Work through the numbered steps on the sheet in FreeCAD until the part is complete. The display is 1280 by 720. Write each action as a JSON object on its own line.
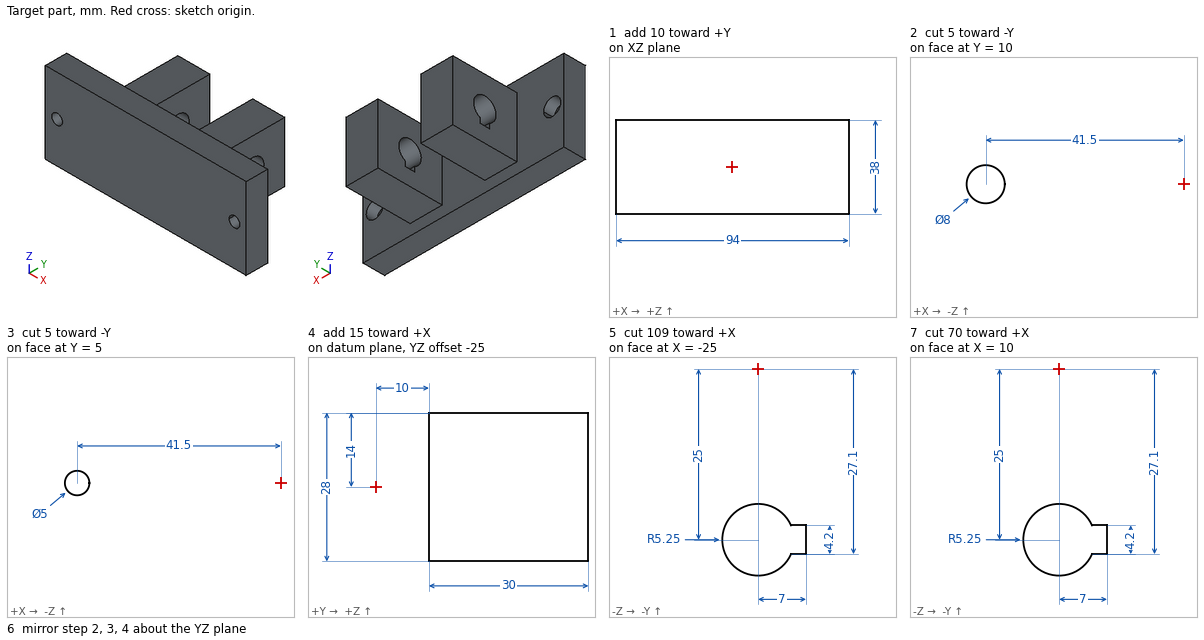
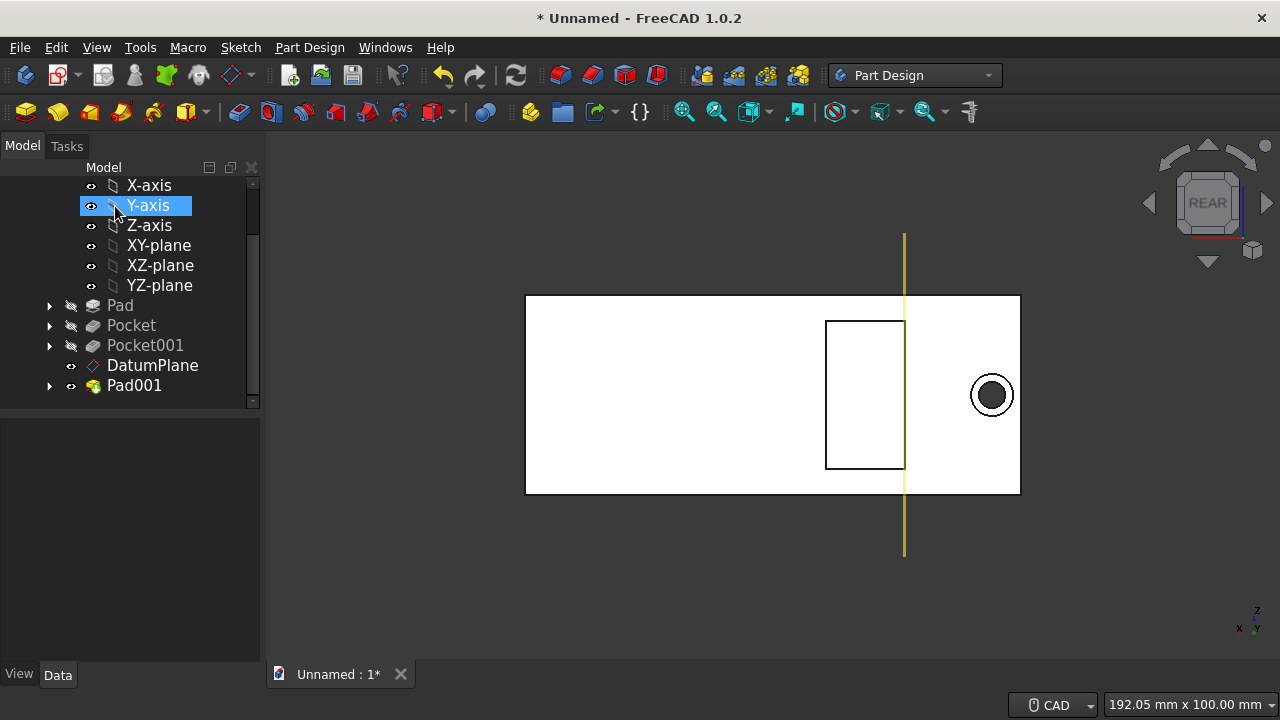
{"action": "left_click", "coordinate": [116, 366]}
{"action": "key", "text": "space"}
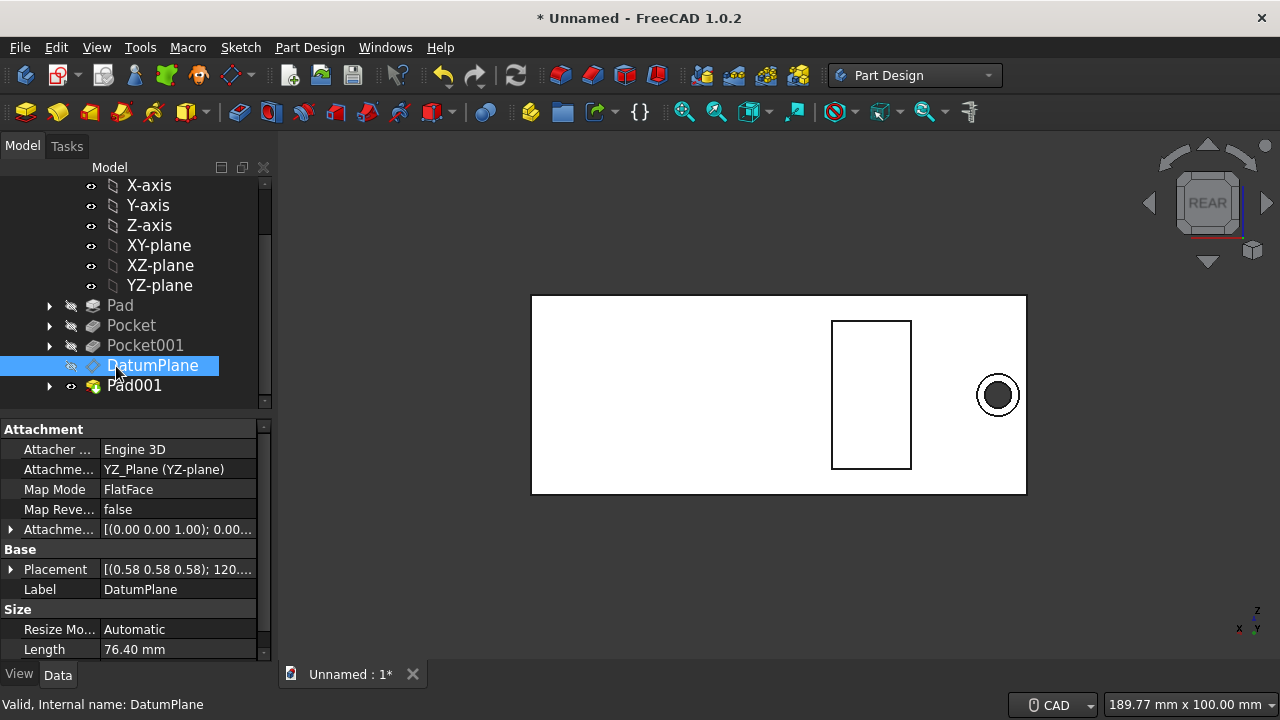
{"action": "key", "text": "6"}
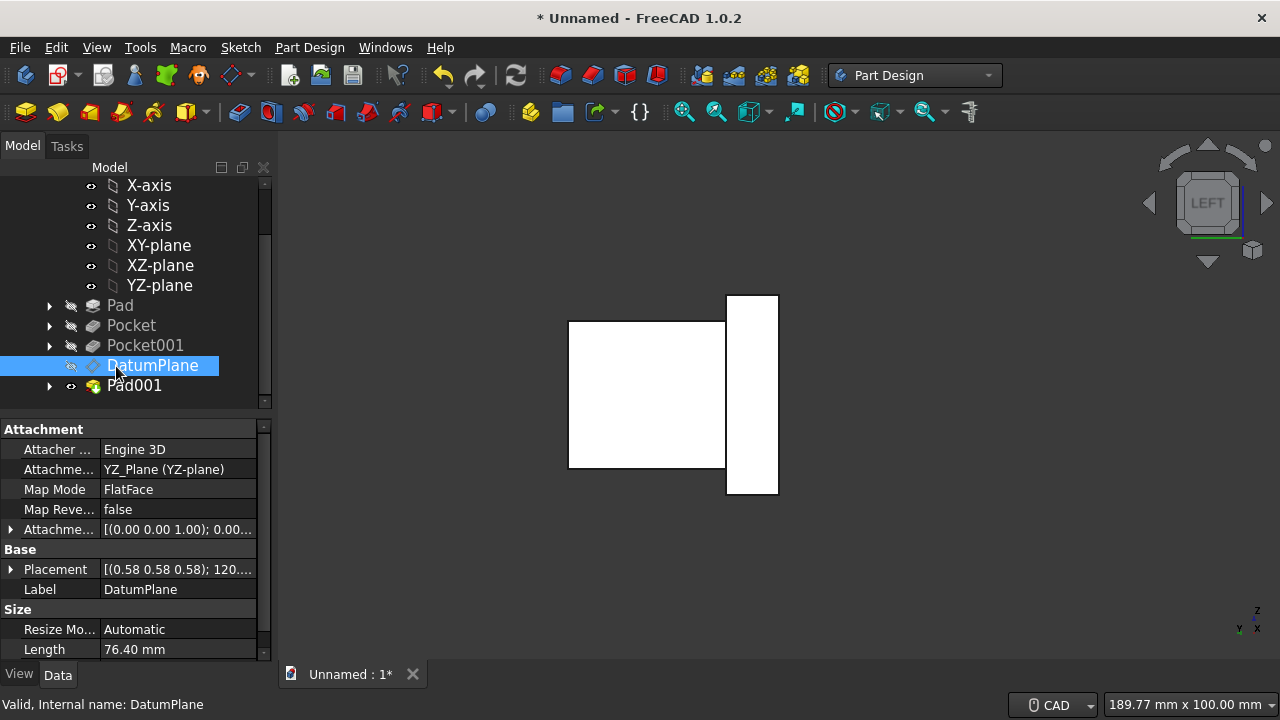
{"action": "left_click", "coordinate": [686, 112]}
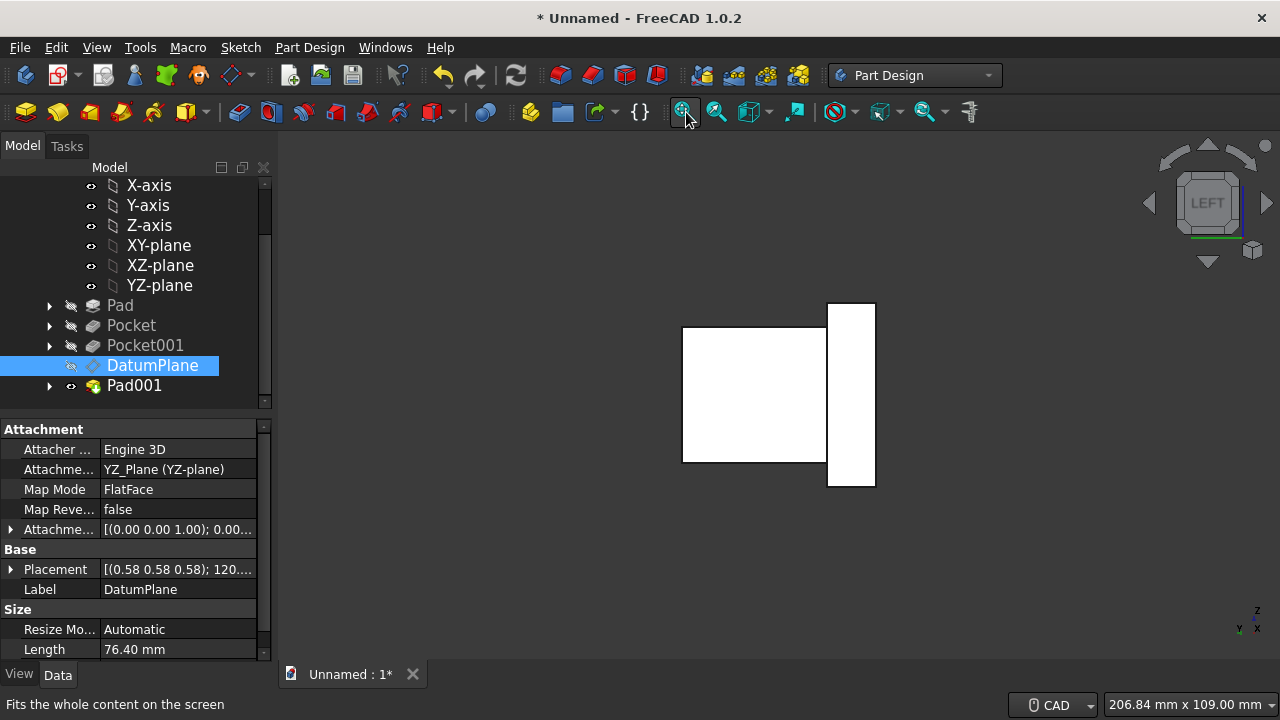
{"action": "left_click", "coordinate": [755, 394]}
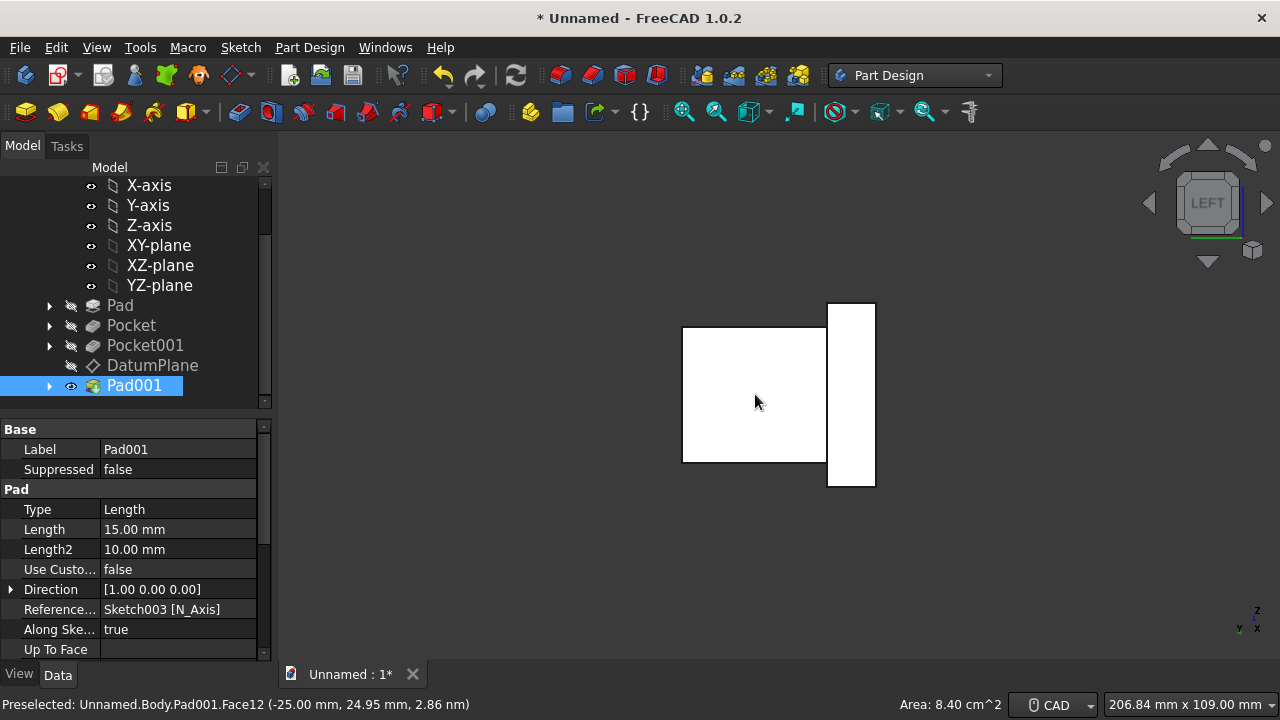
{"action": "left_click", "coordinate": [58, 76]}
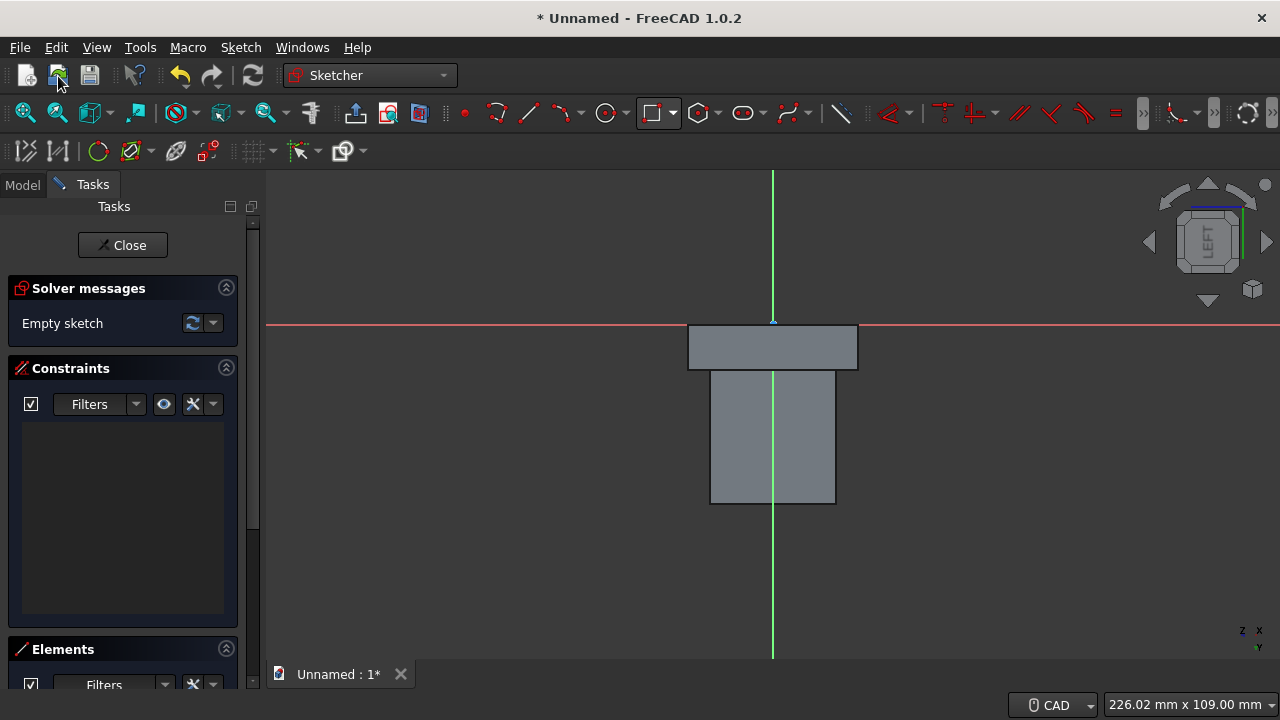
{"action": "scroll", "coordinate": [819, 369], "scroll_direction": "up", "scroll_amount": 5}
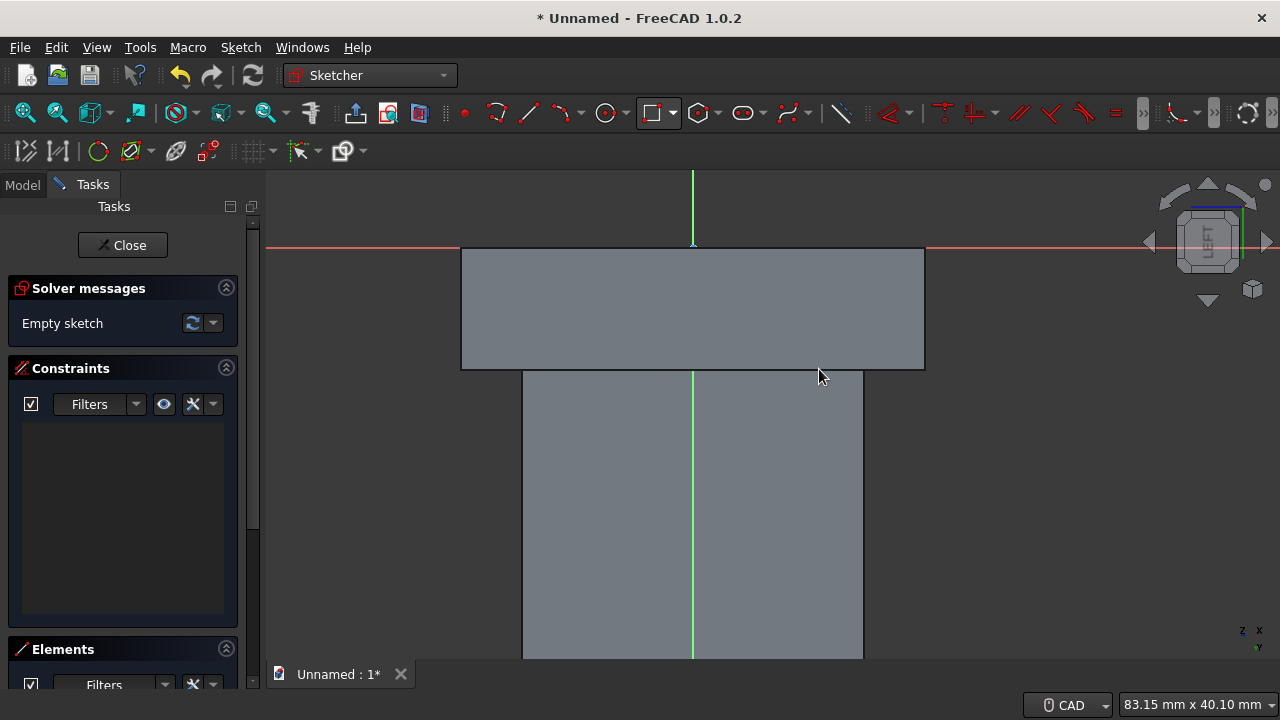
{"action": "left_click", "coordinate": [498, 114]}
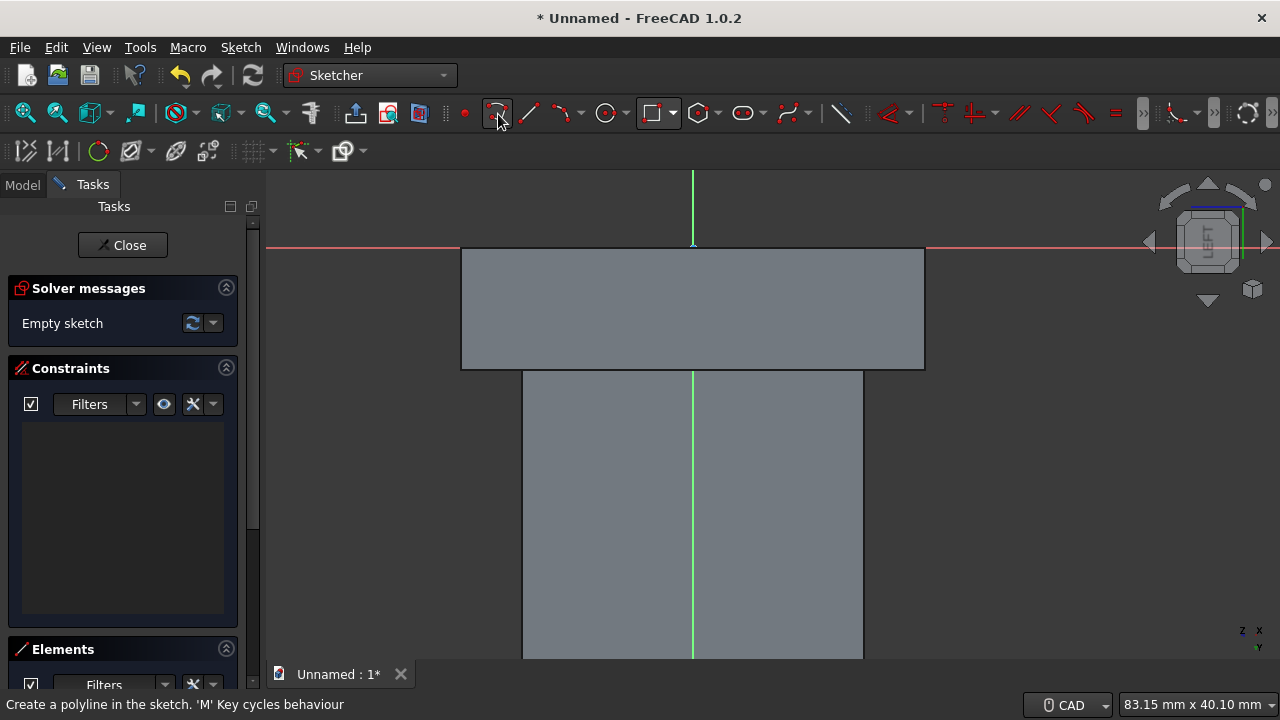
{"action": "left_click", "coordinate": [752, 579]}
{"action": "left_click", "coordinate": [778, 579]}
{"action": "left_click", "coordinate": [778, 527]}
{"action": "left_click", "coordinate": [752, 527]}
{"action": "right_click", "coordinate": [752, 527]}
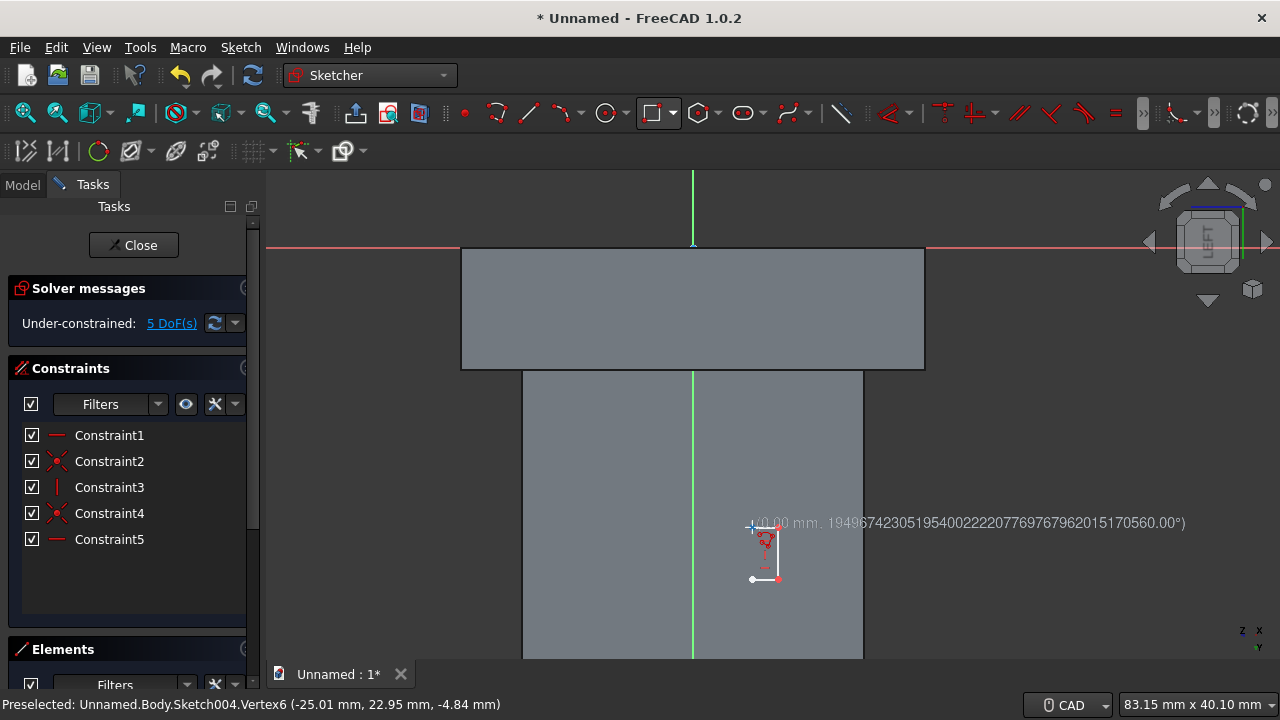
{"action": "left_click", "coordinate": [562, 114]}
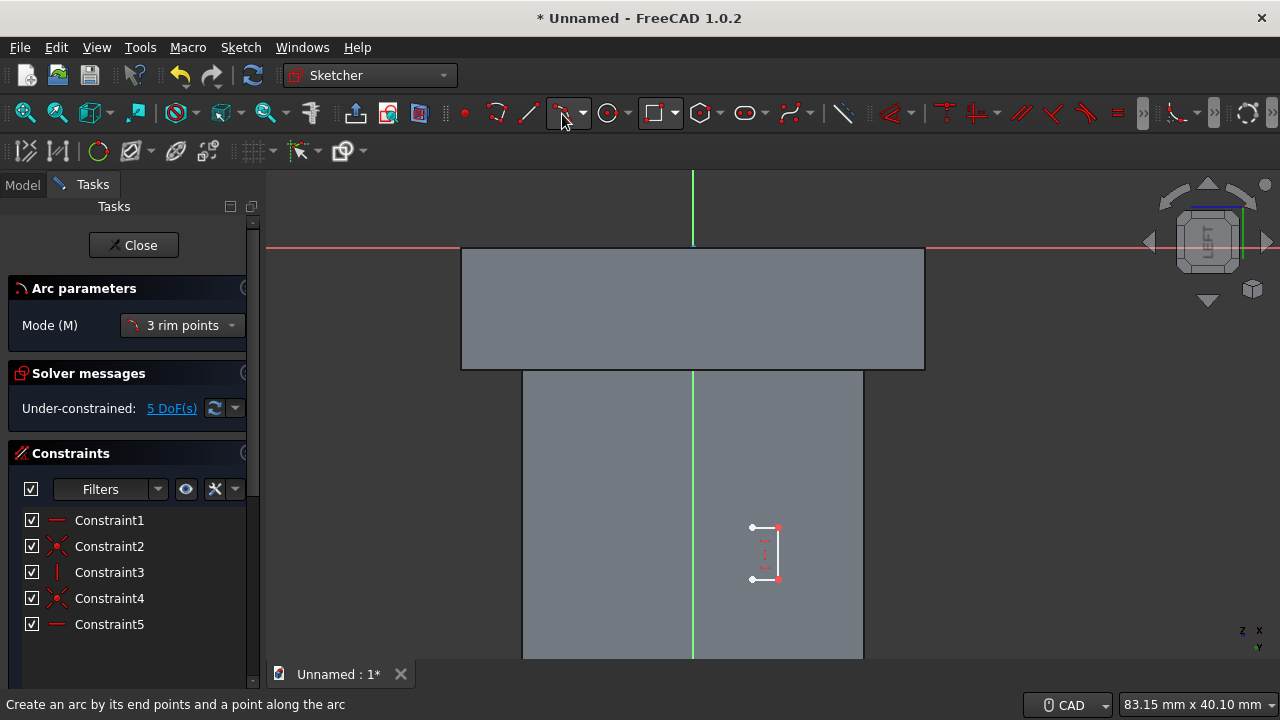
{"action": "left_click", "coordinate": [752, 528]}
{"action": "left_click", "coordinate": [752, 580]}
{"action": "left_click", "coordinate": [629, 553]}
{"action": "key", "text": "Escape"}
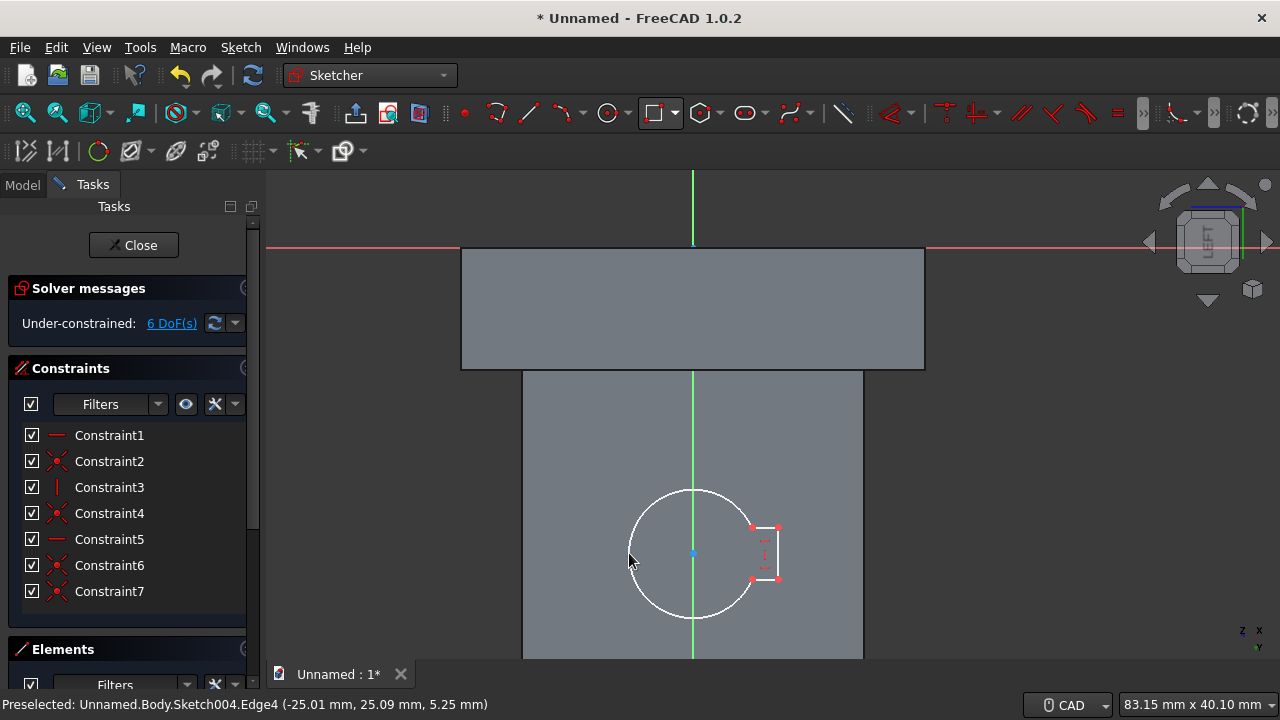
{"action": "left_click", "coordinate": [693, 554]}